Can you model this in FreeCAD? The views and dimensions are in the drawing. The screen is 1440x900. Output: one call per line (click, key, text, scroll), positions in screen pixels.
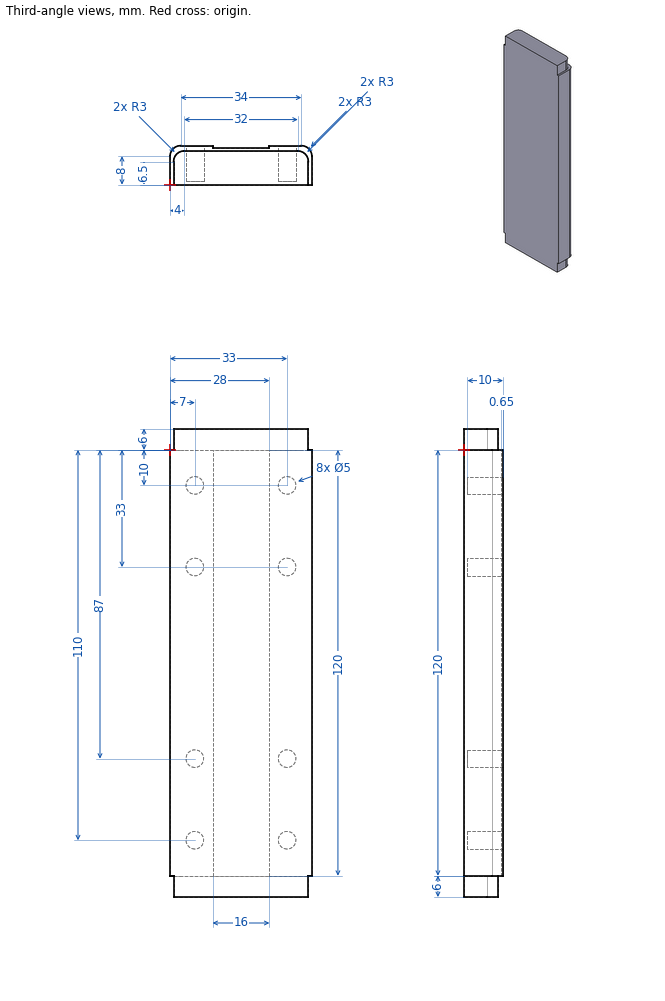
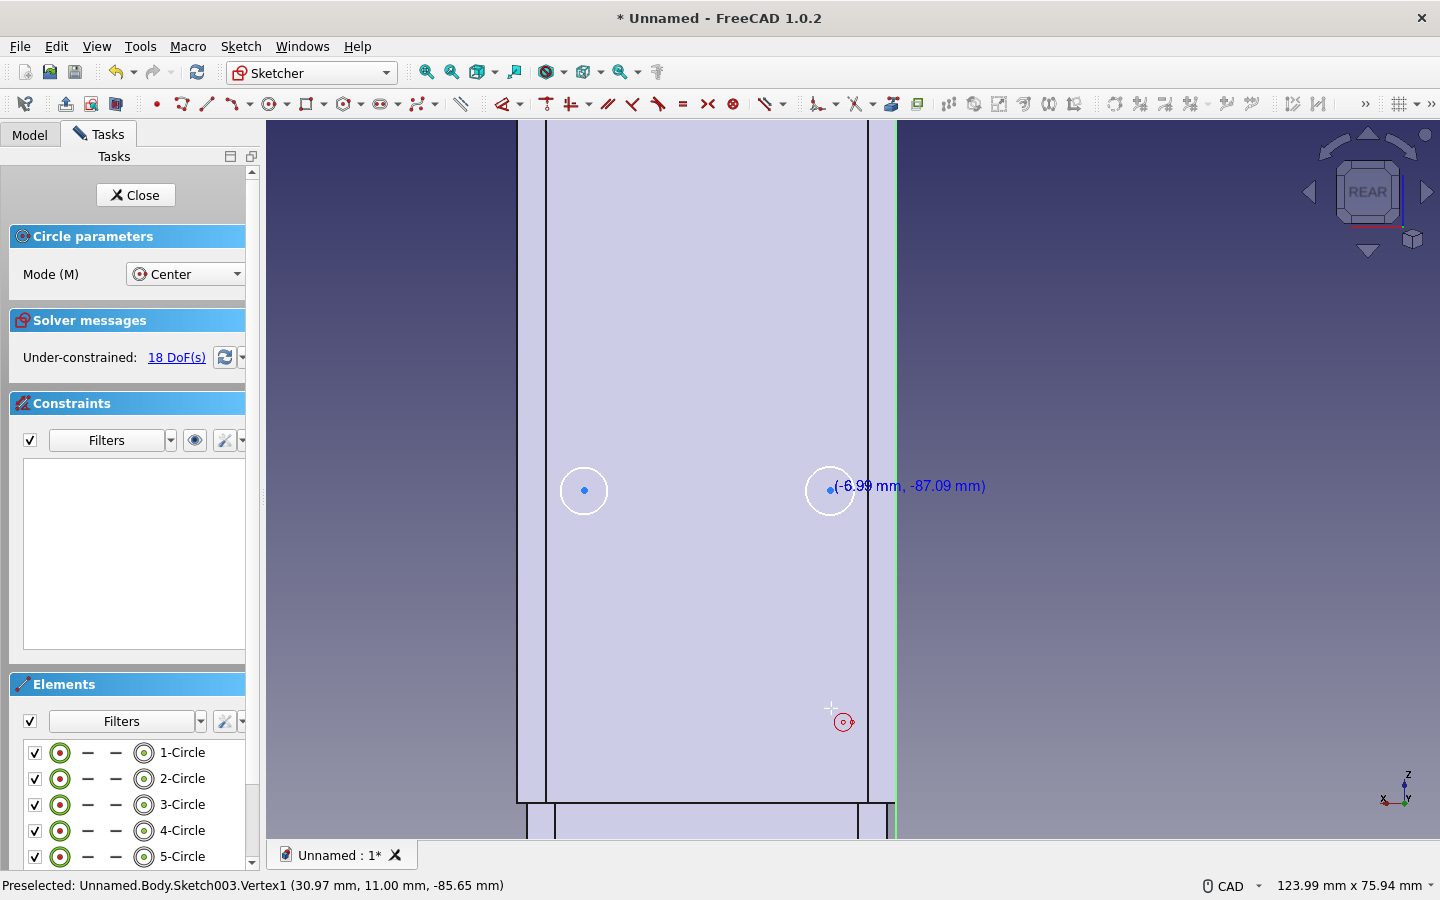
click(830, 708)
click(847, 691)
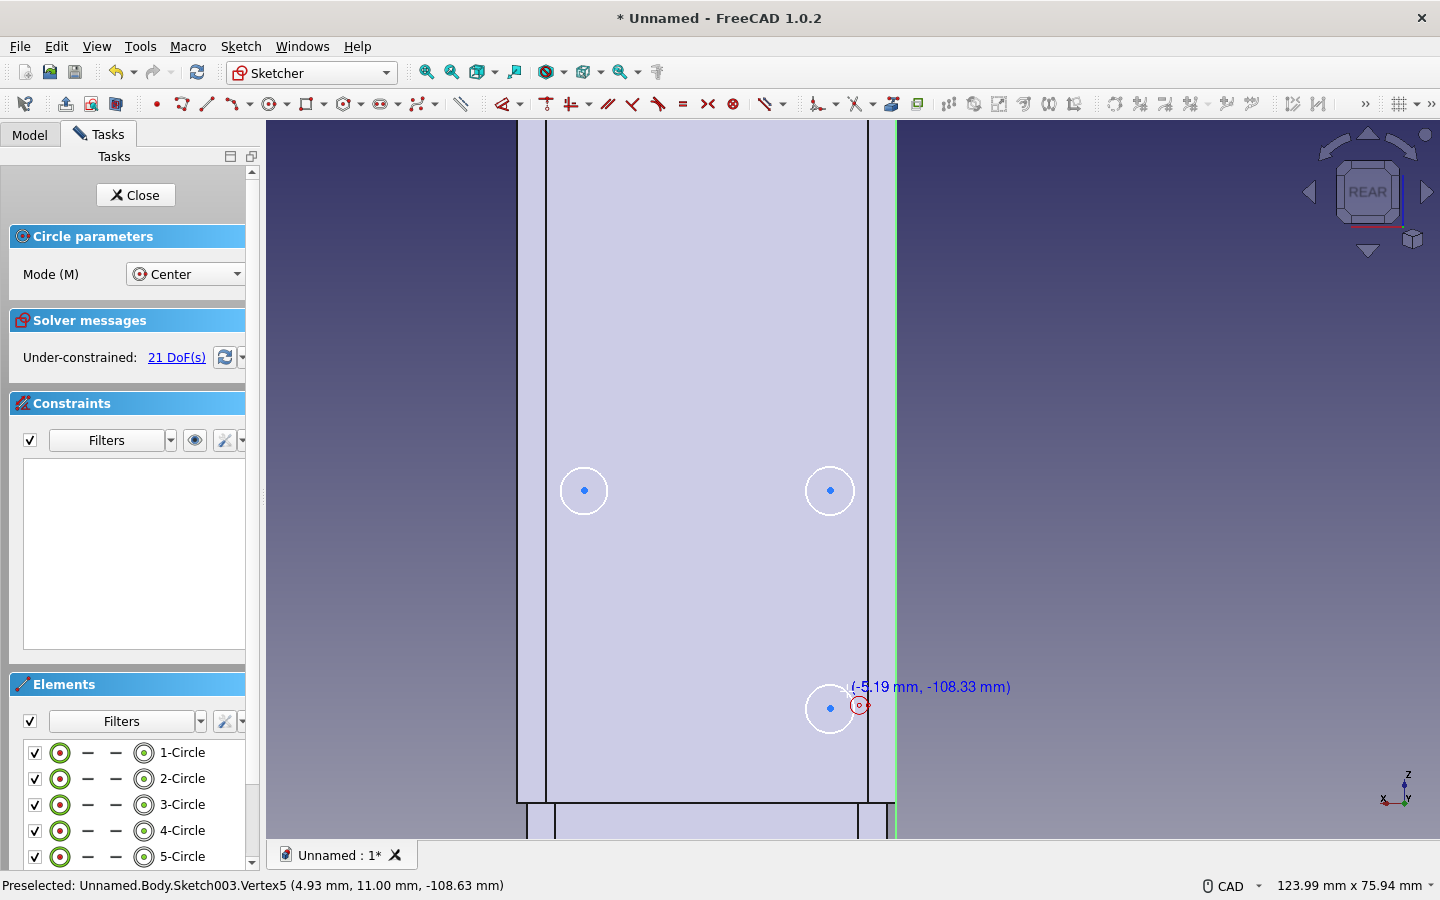
click(584, 708)
click(600, 691)
key(Escape)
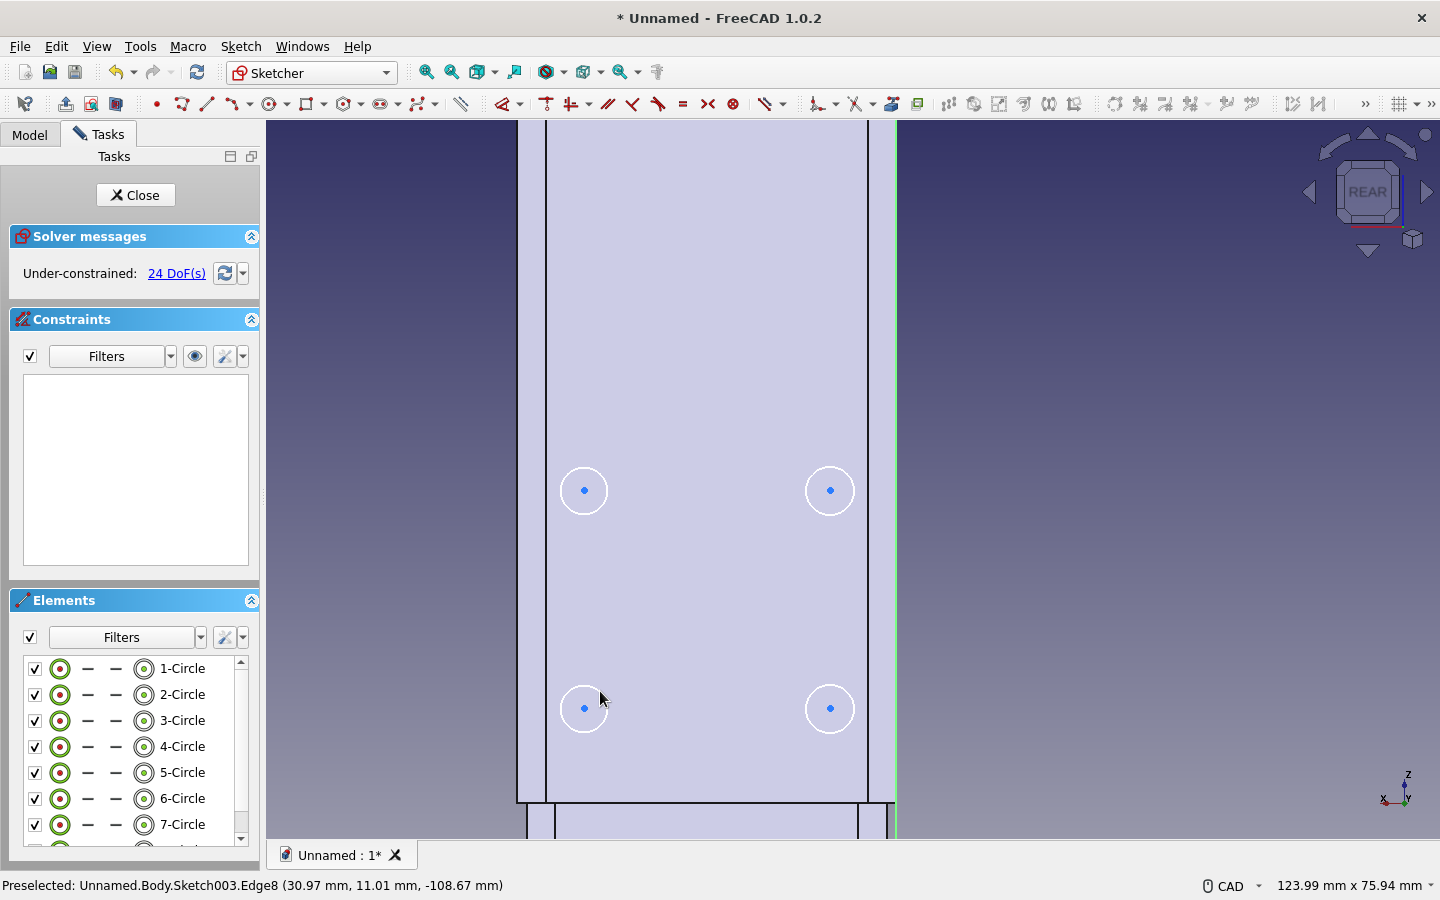
scroll(831, 708, down, 4)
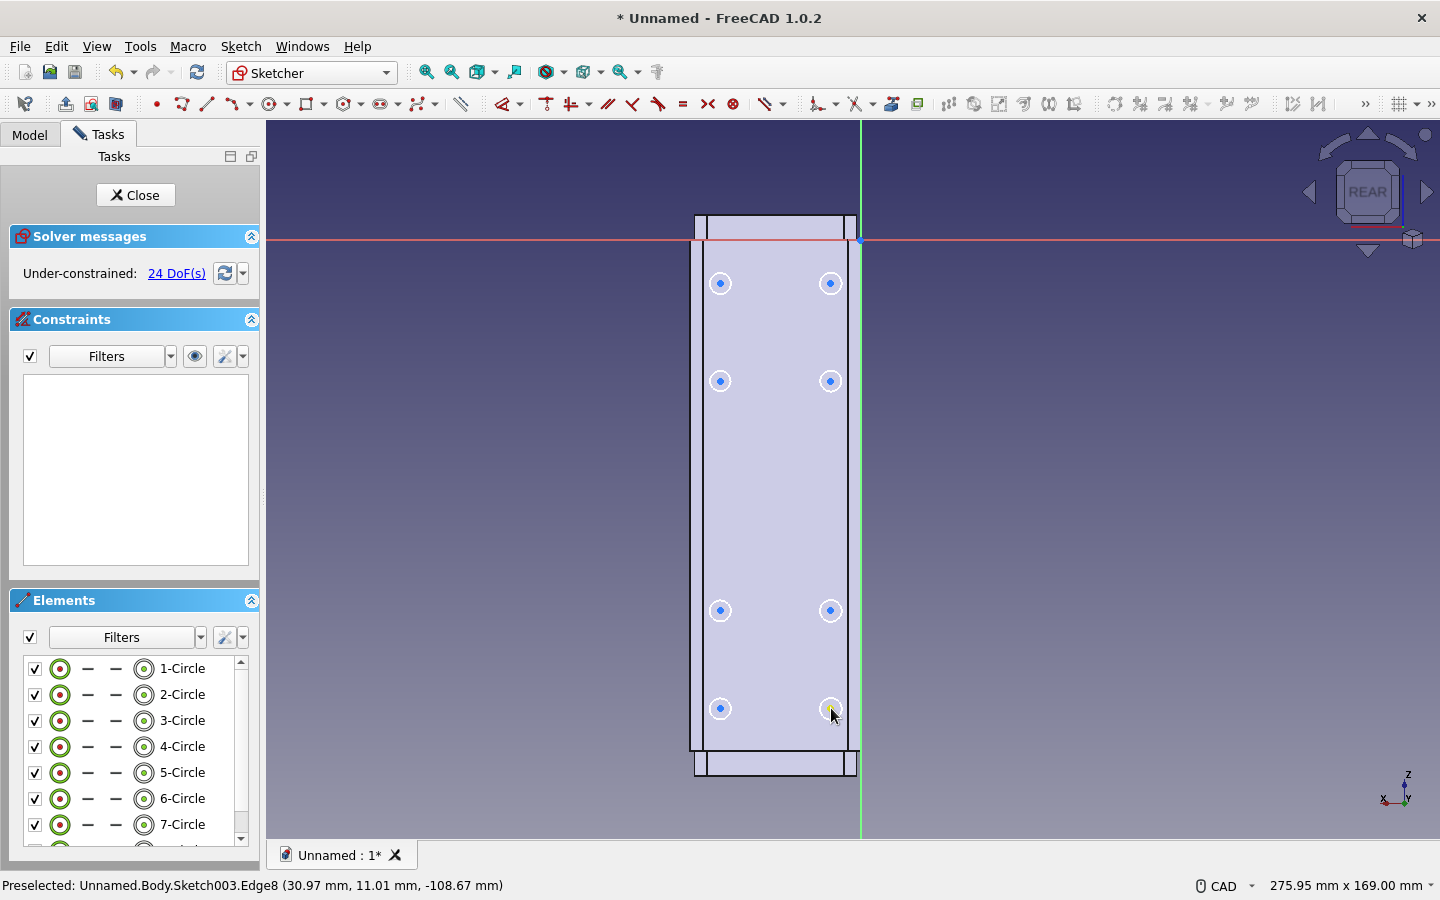
scroll(728, 276, up, 2)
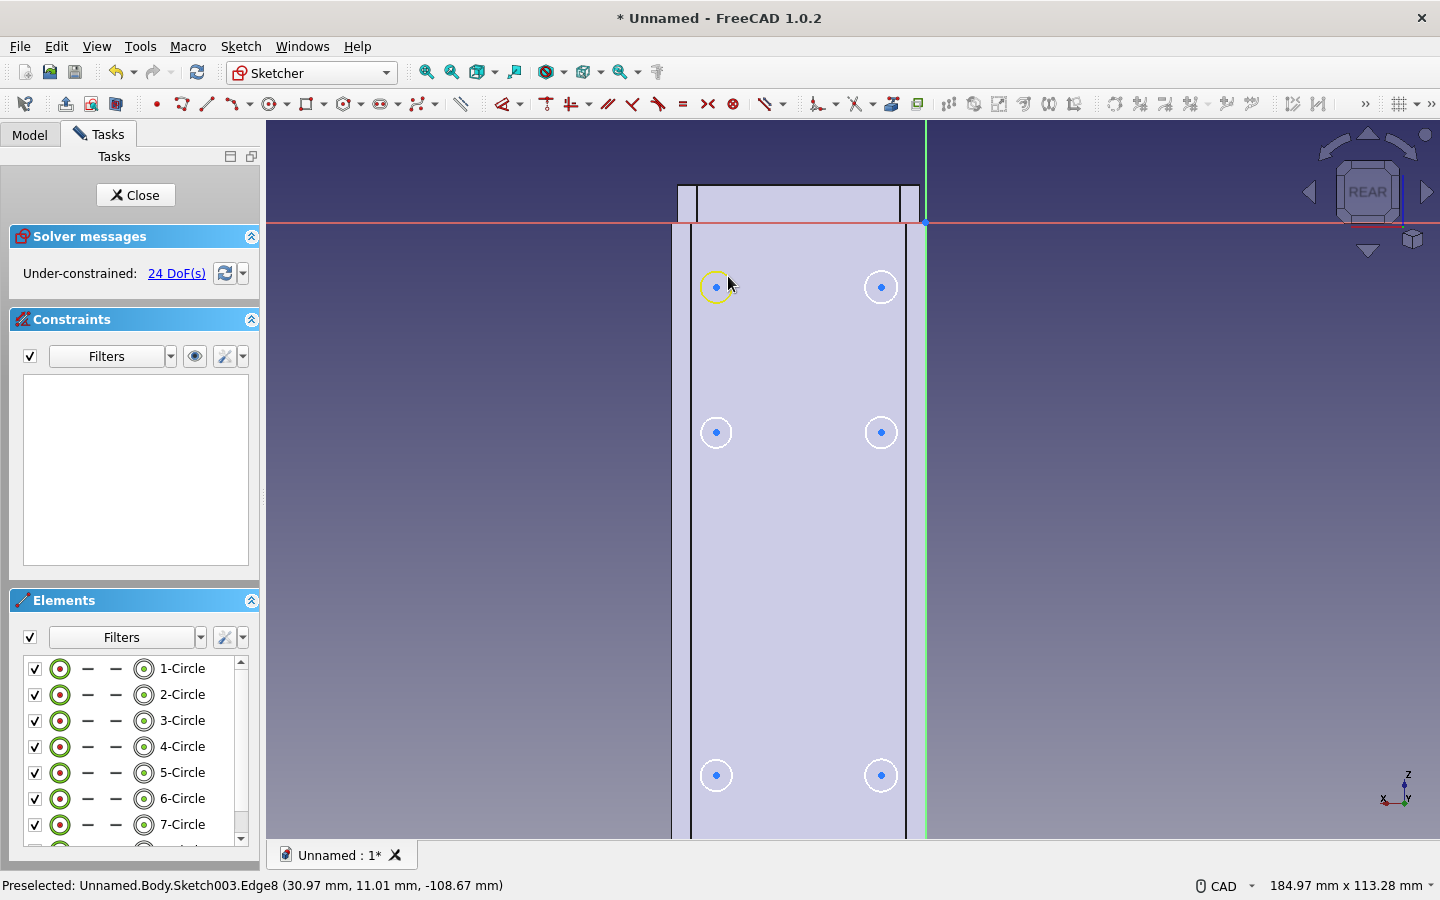
click(727, 276)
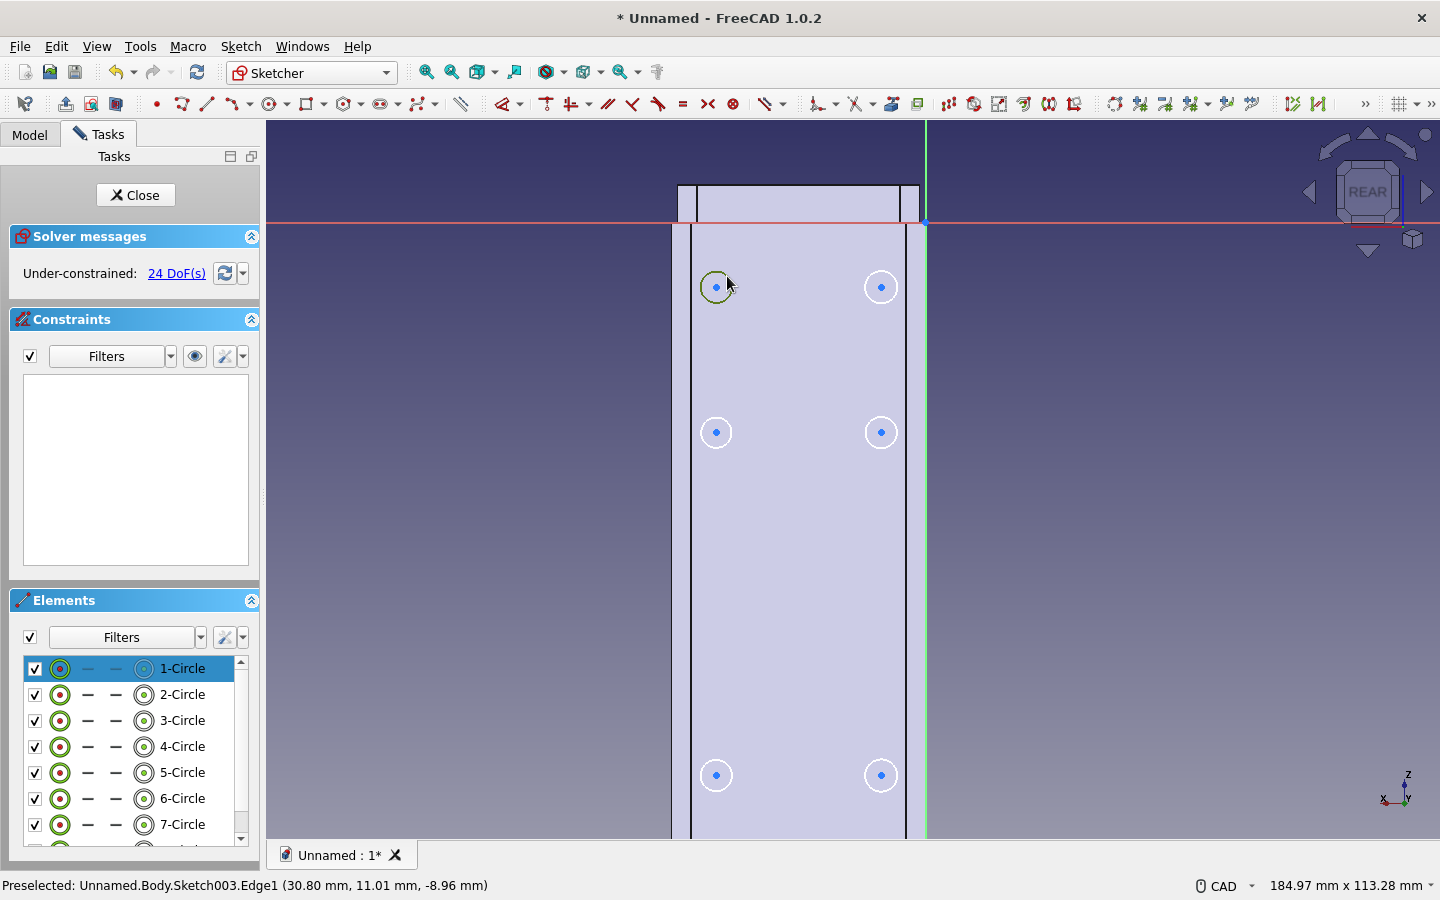
click(893, 276)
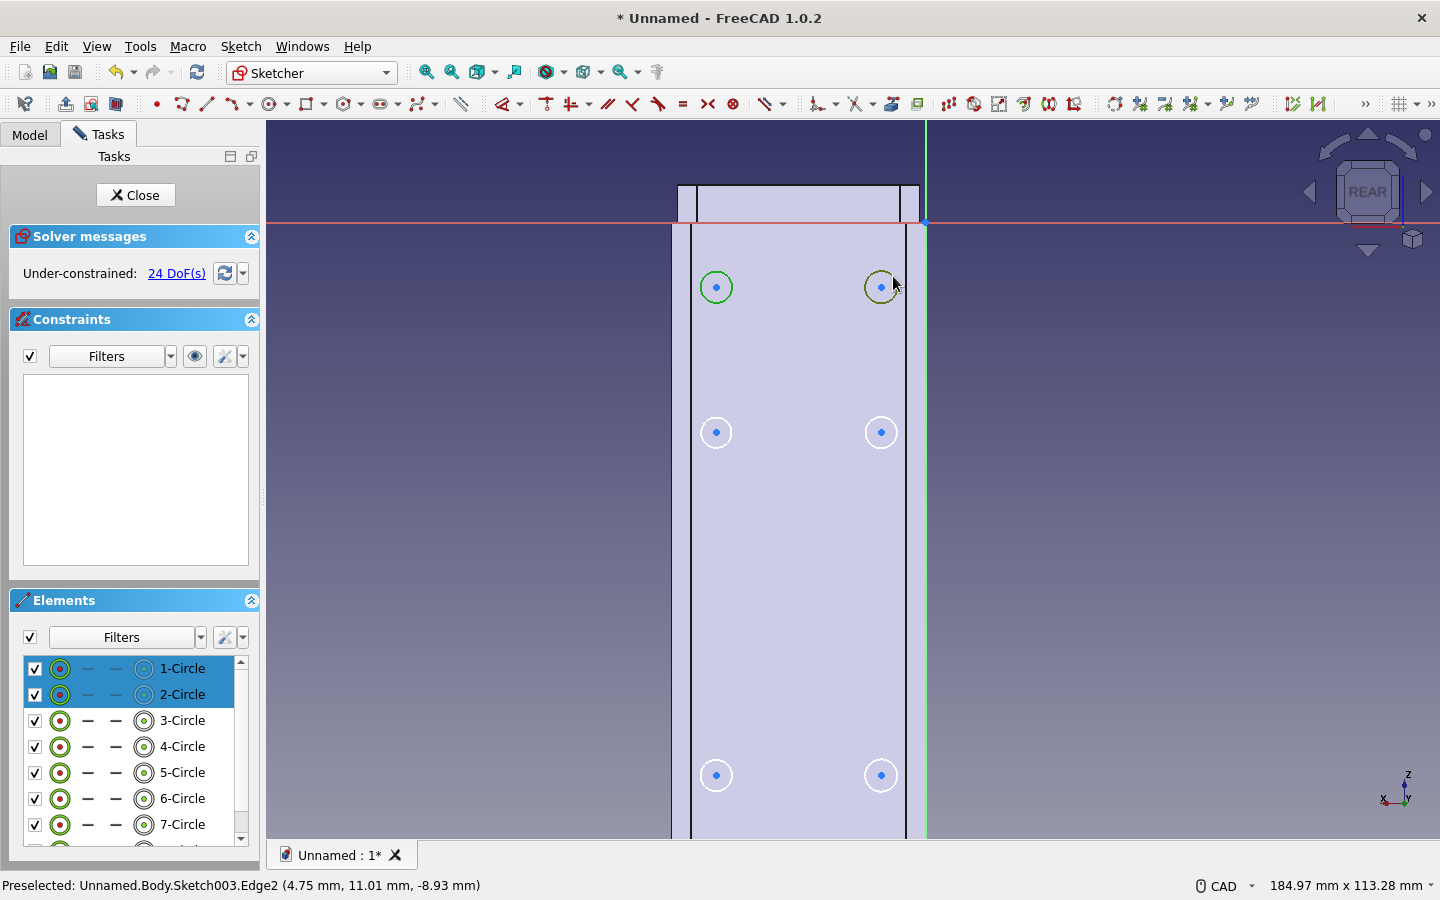
click(727, 422)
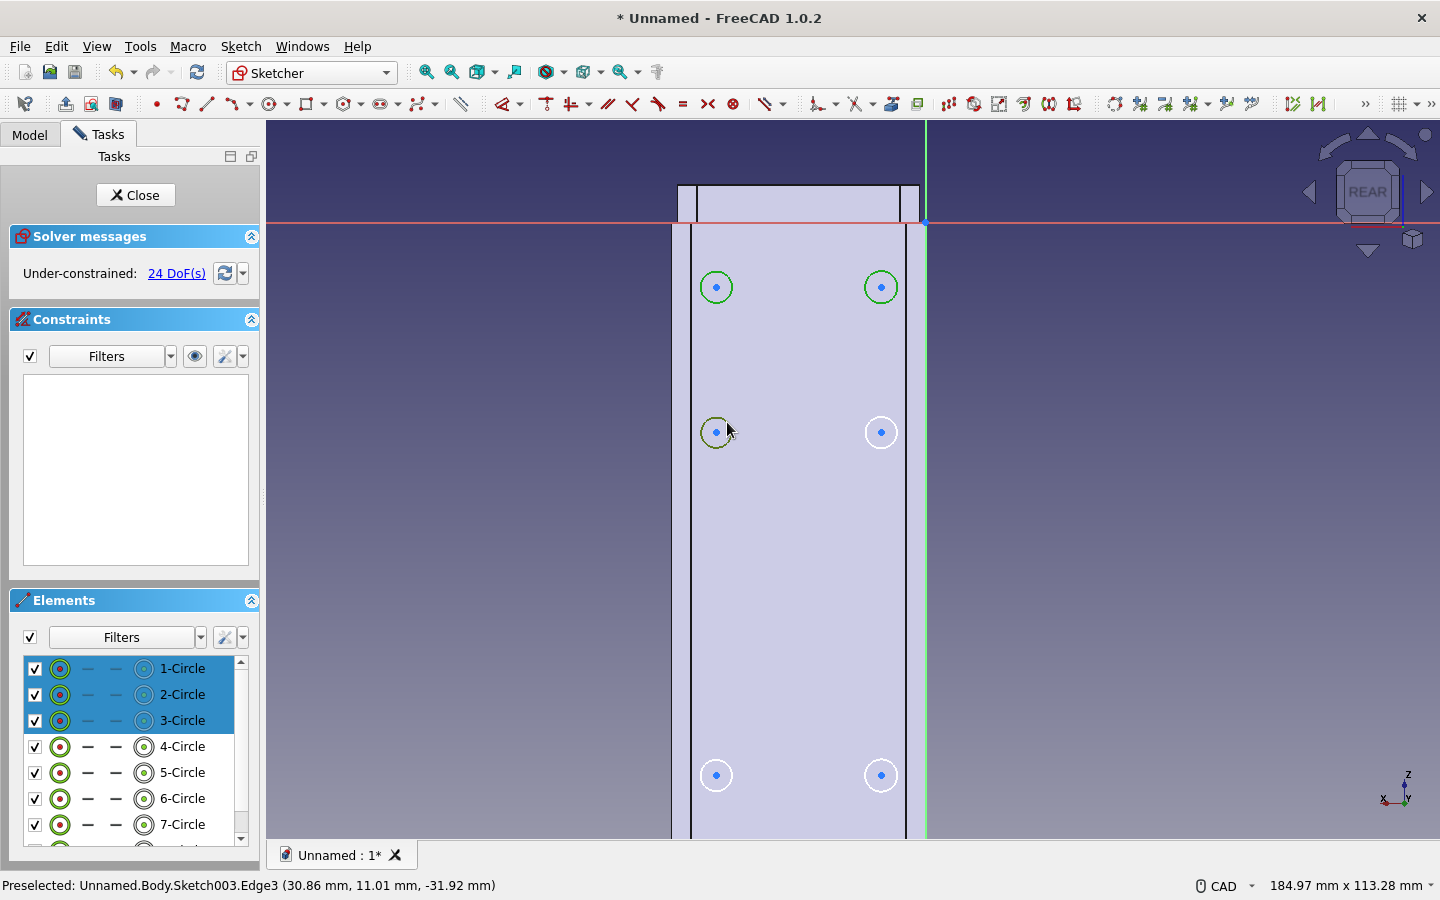
click(892, 422)